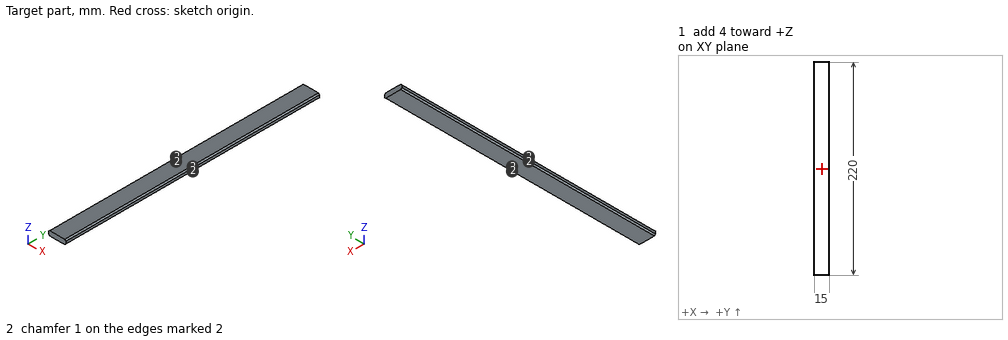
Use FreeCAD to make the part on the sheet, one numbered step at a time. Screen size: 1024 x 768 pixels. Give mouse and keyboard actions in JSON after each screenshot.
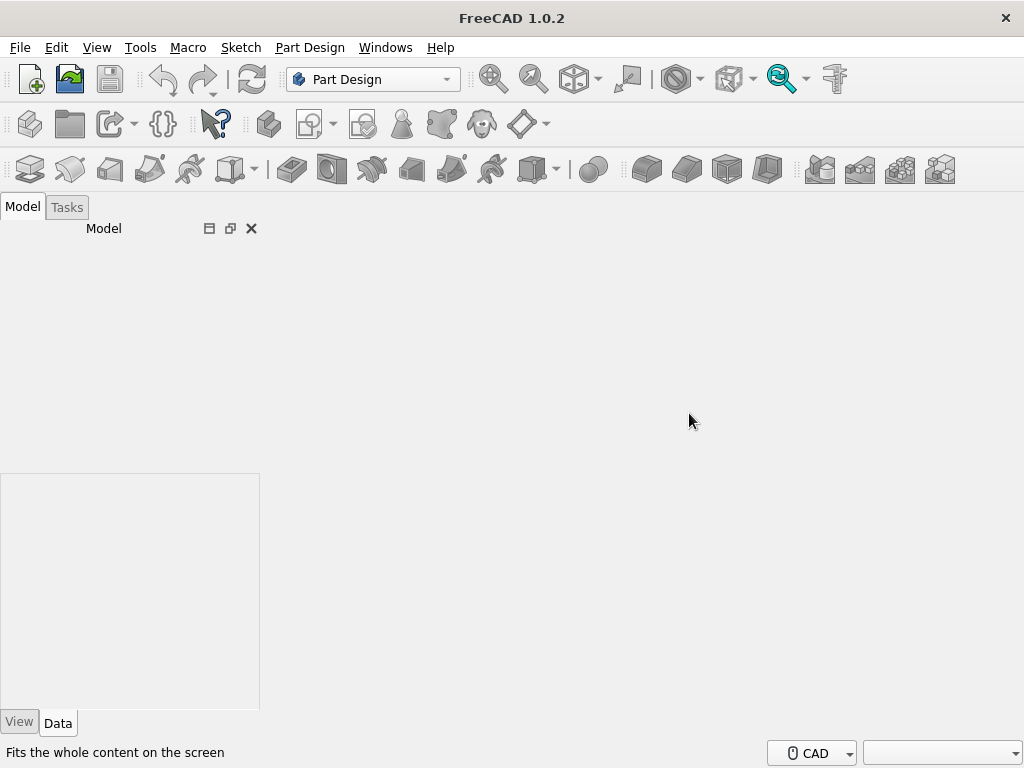
{"action": "key", "text": "ctrl+n"}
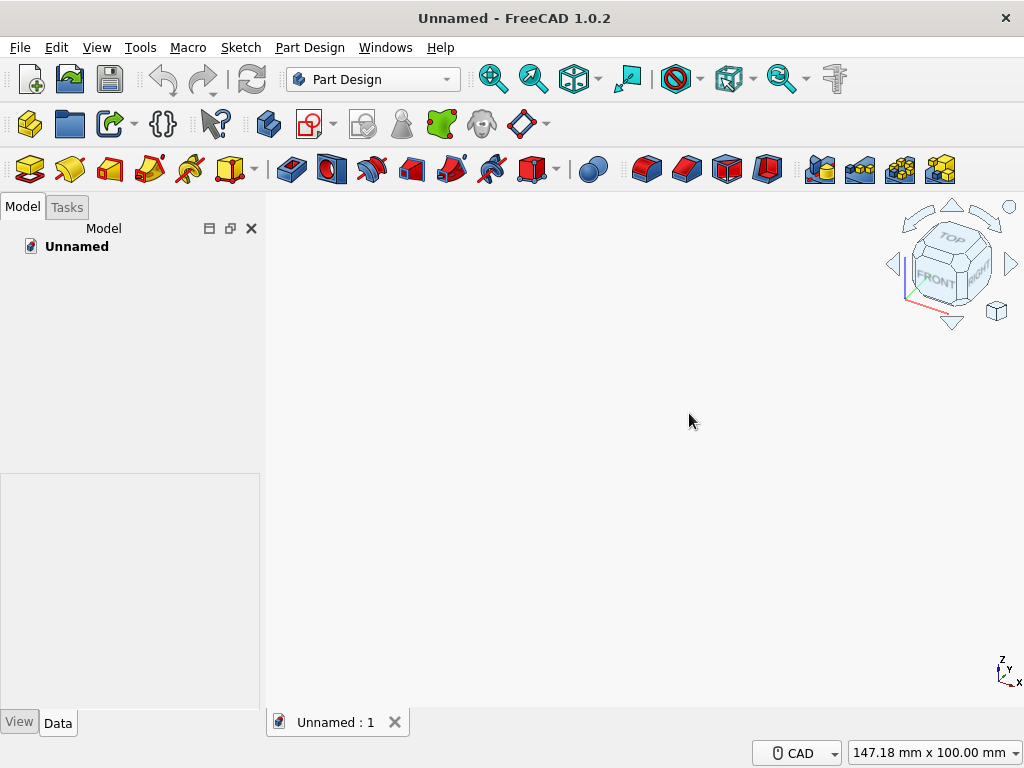
{"action": "left_click", "coordinate": [310, 124]}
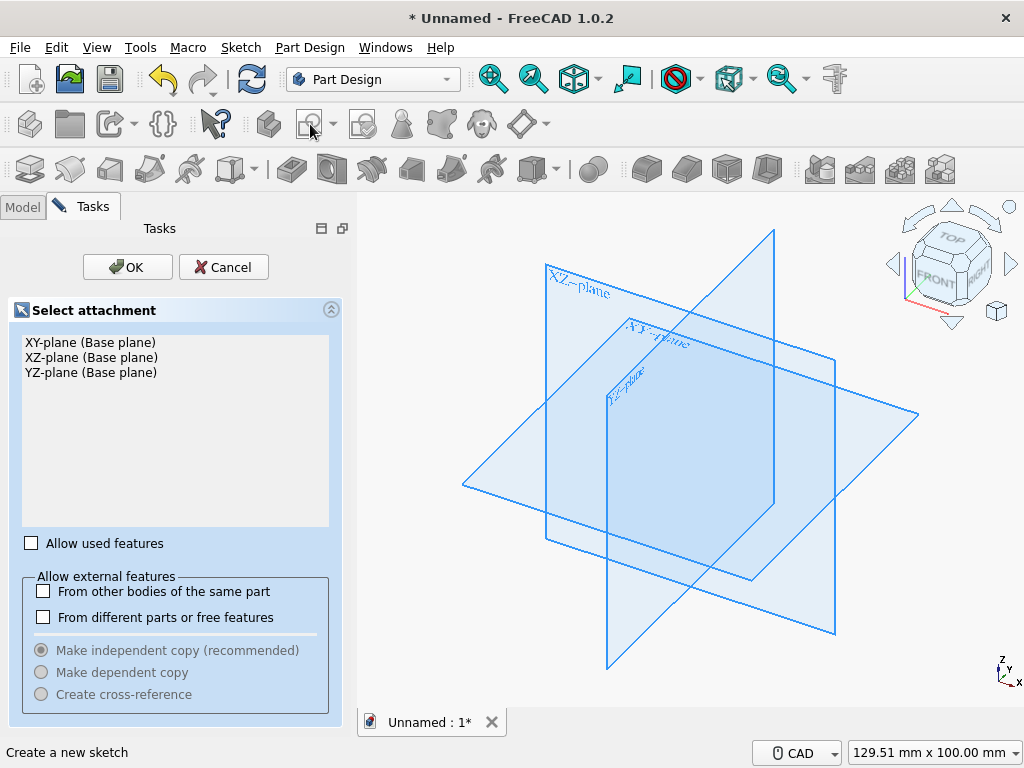
{"action": "left_click", "coordinate": [82, 342]}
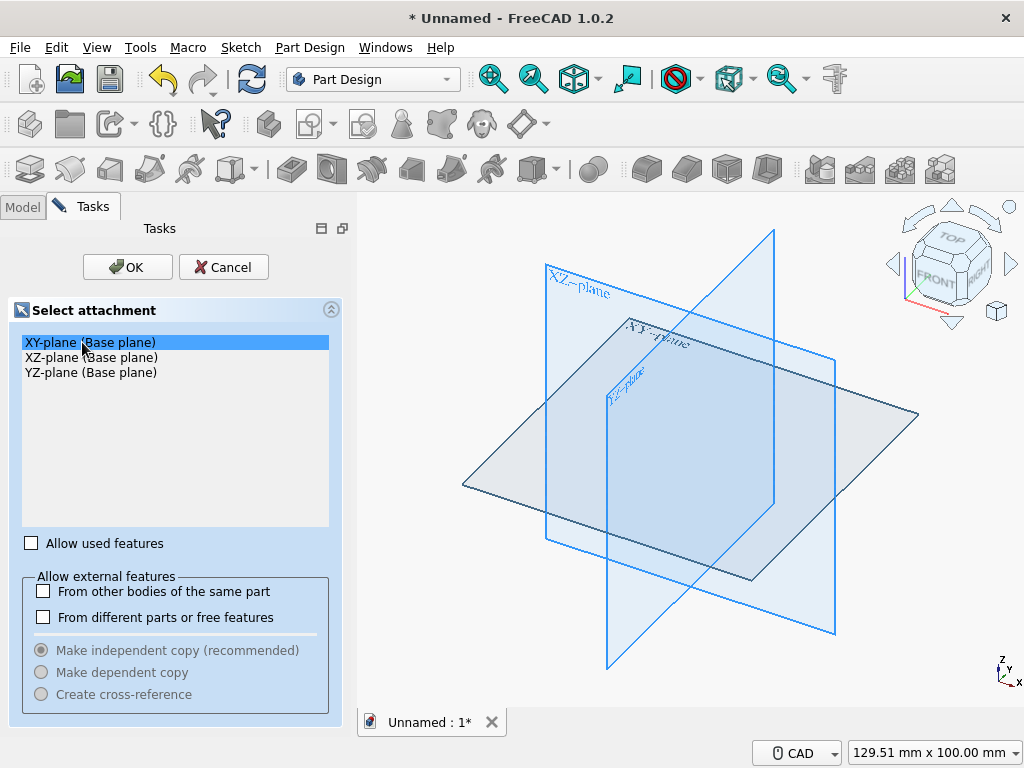
{"action": "left_click", "coordinate": [128, 267]}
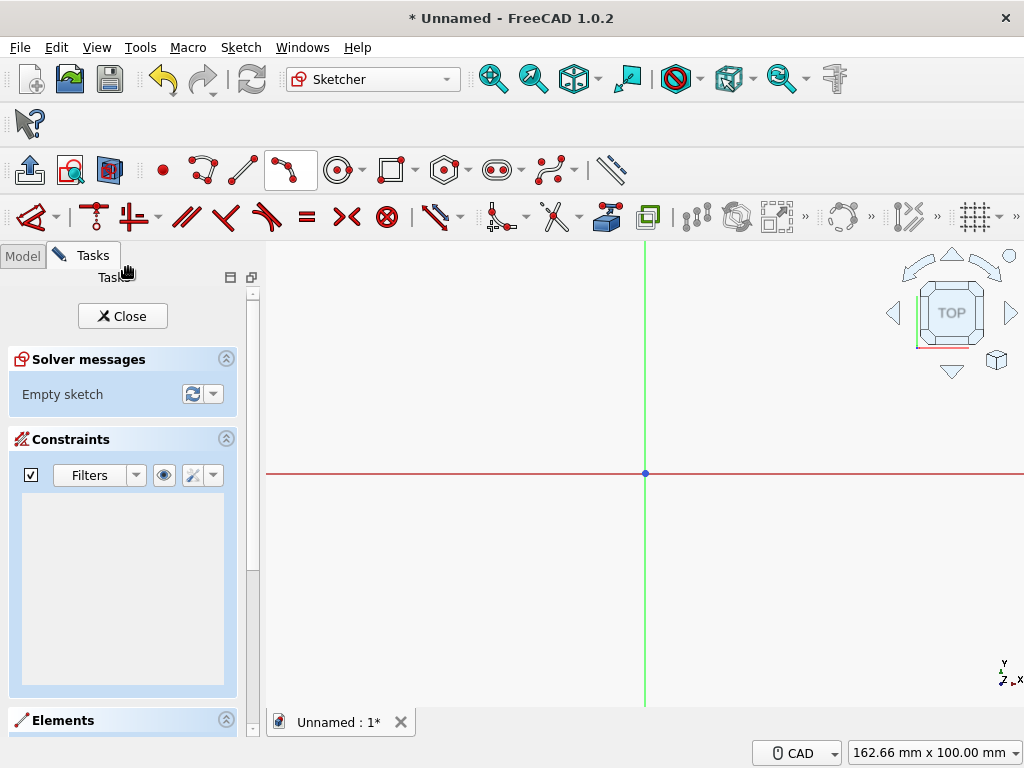
{"action": "scroll", "coordinate": [547, 474], "scroll_direction": "down", "scroll_amount": 6}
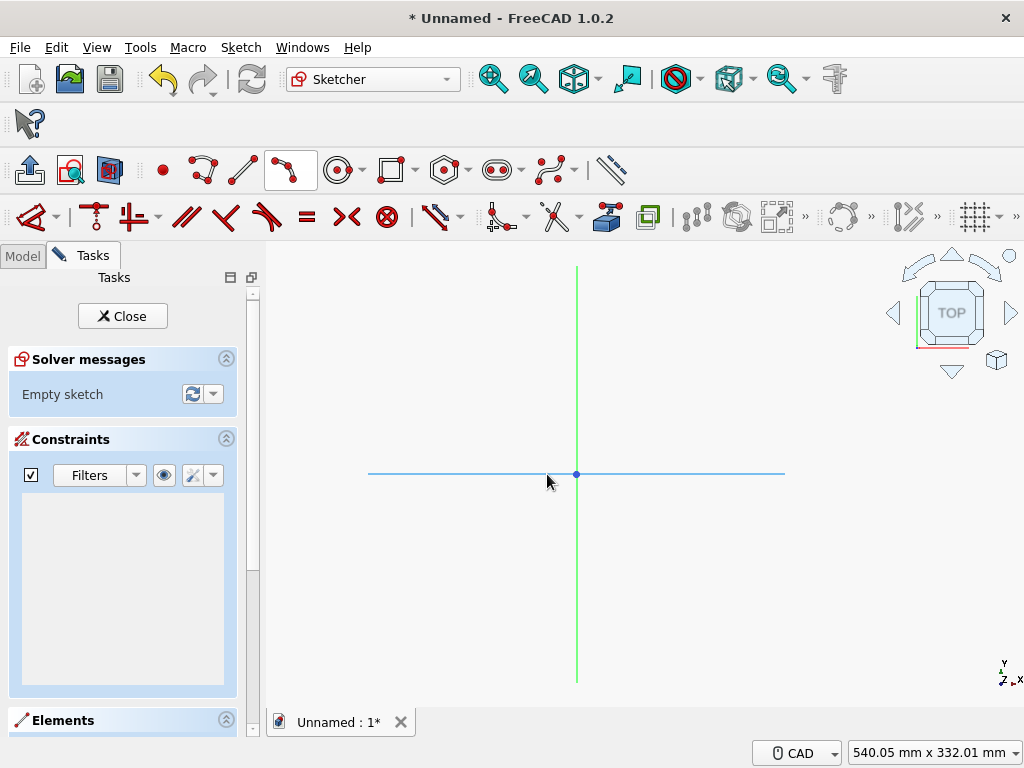
{"action": "key", "text": "g v"}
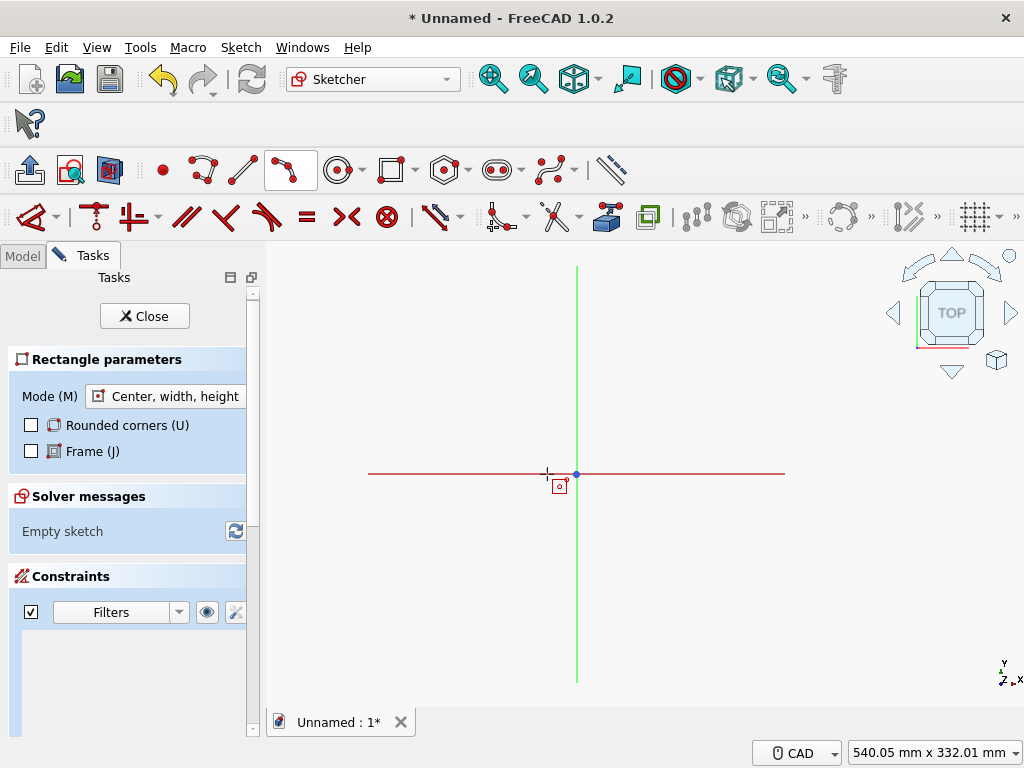
{"action": "scroll", "coordinate": [577, 474], "scroll_direction": "up", "scroll_amount": 3}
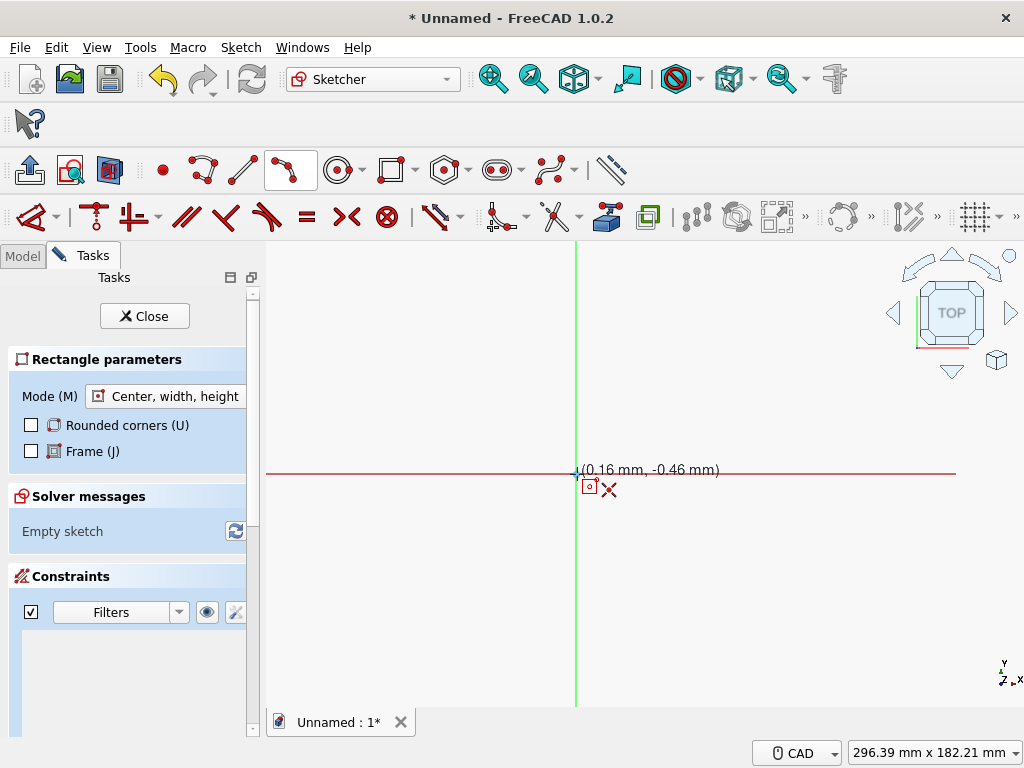
{"action": "left_click", "coordinate": [576, 474]}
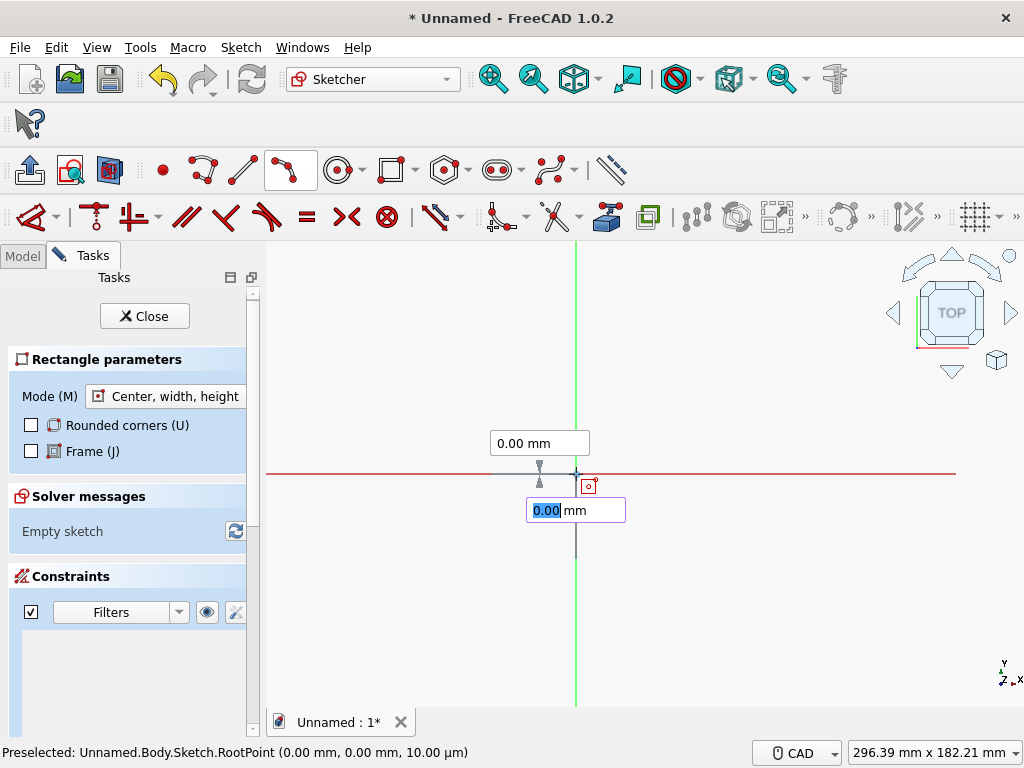
{"action": "scroll", "coordinate": [577, 474], "scroll_direction": "down", "scroll_amount": 3}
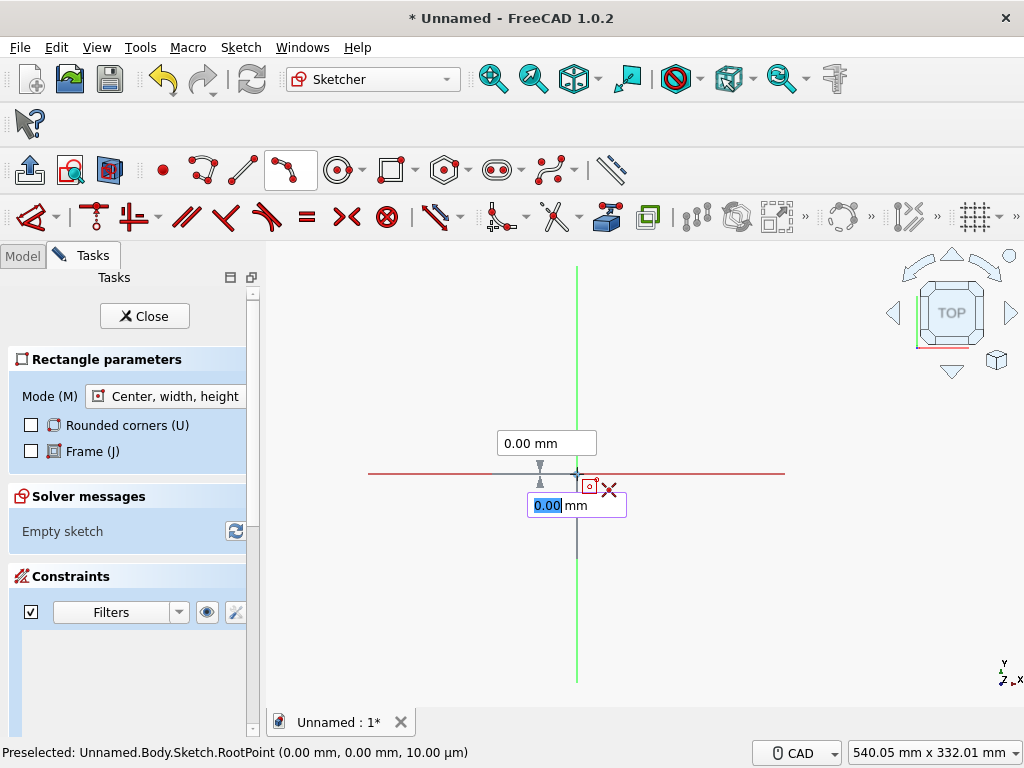
{"action": "scroll", "coordinate": [587, 320], "scroll_direction": "up", "scroll_amount": 3}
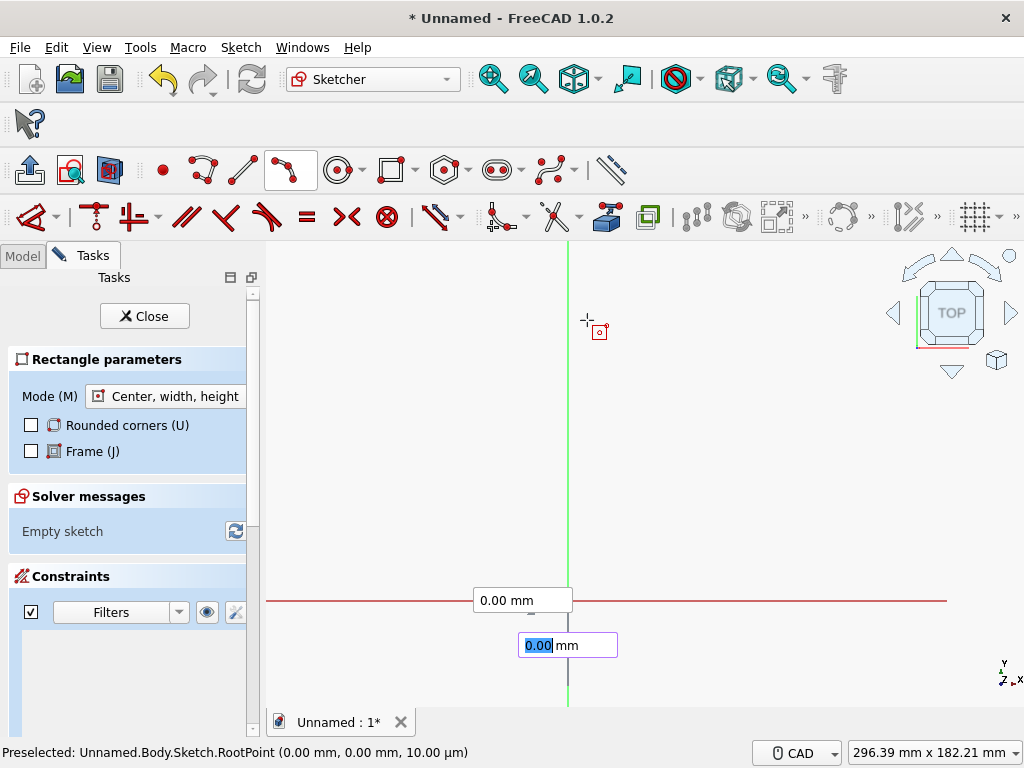
{"action": "left_click", "coordinate": [587, 320]}
{"action": "key", "text": "Escape"}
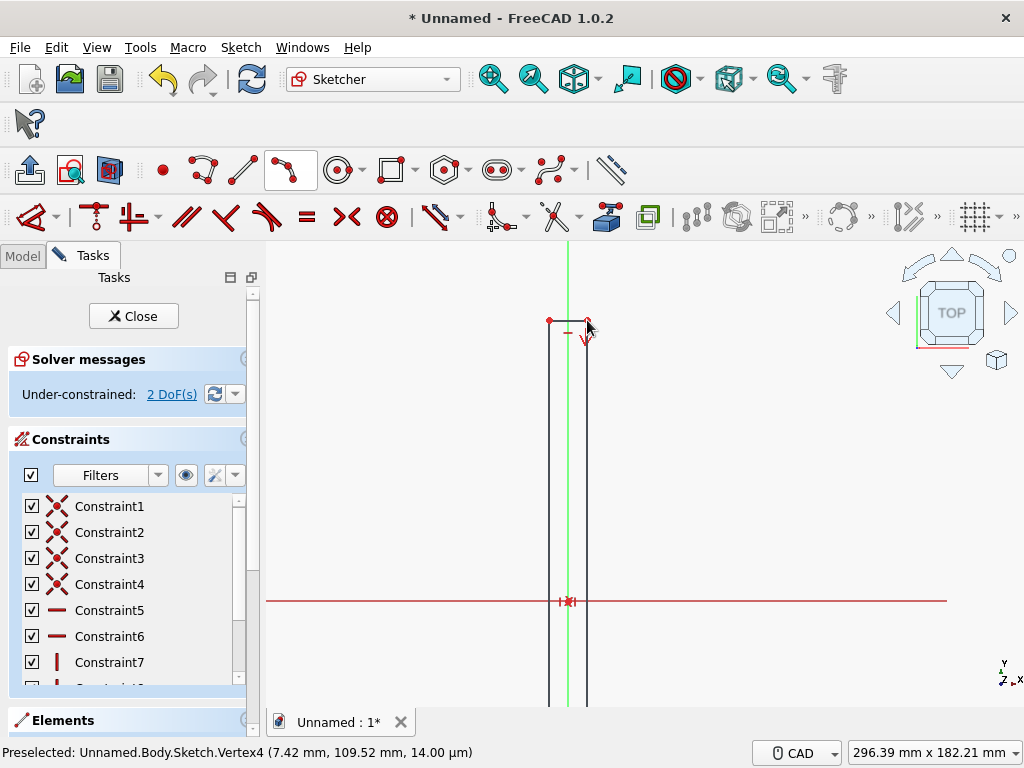
{"action": "key", "text": "d"}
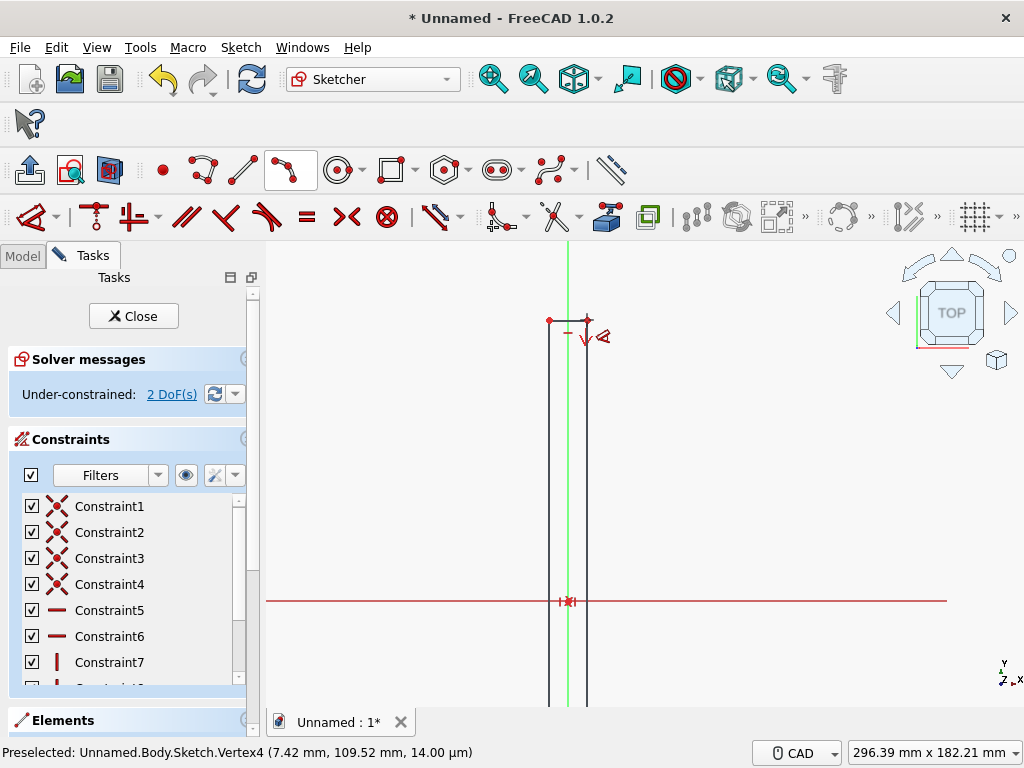
{"action": "scroll", "coordinate": [587, 319], "scroll_direction": "down", "scroll_amount": 3}